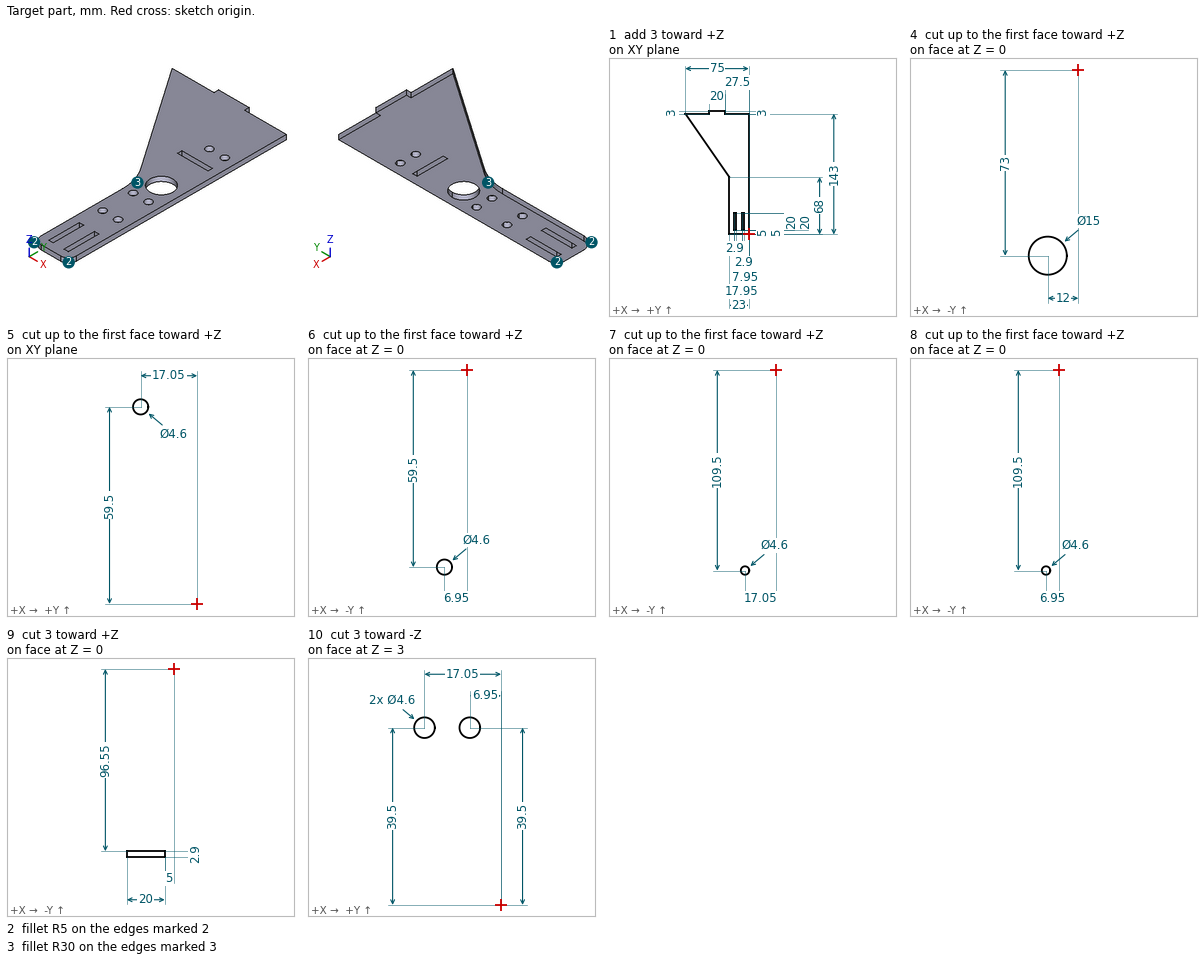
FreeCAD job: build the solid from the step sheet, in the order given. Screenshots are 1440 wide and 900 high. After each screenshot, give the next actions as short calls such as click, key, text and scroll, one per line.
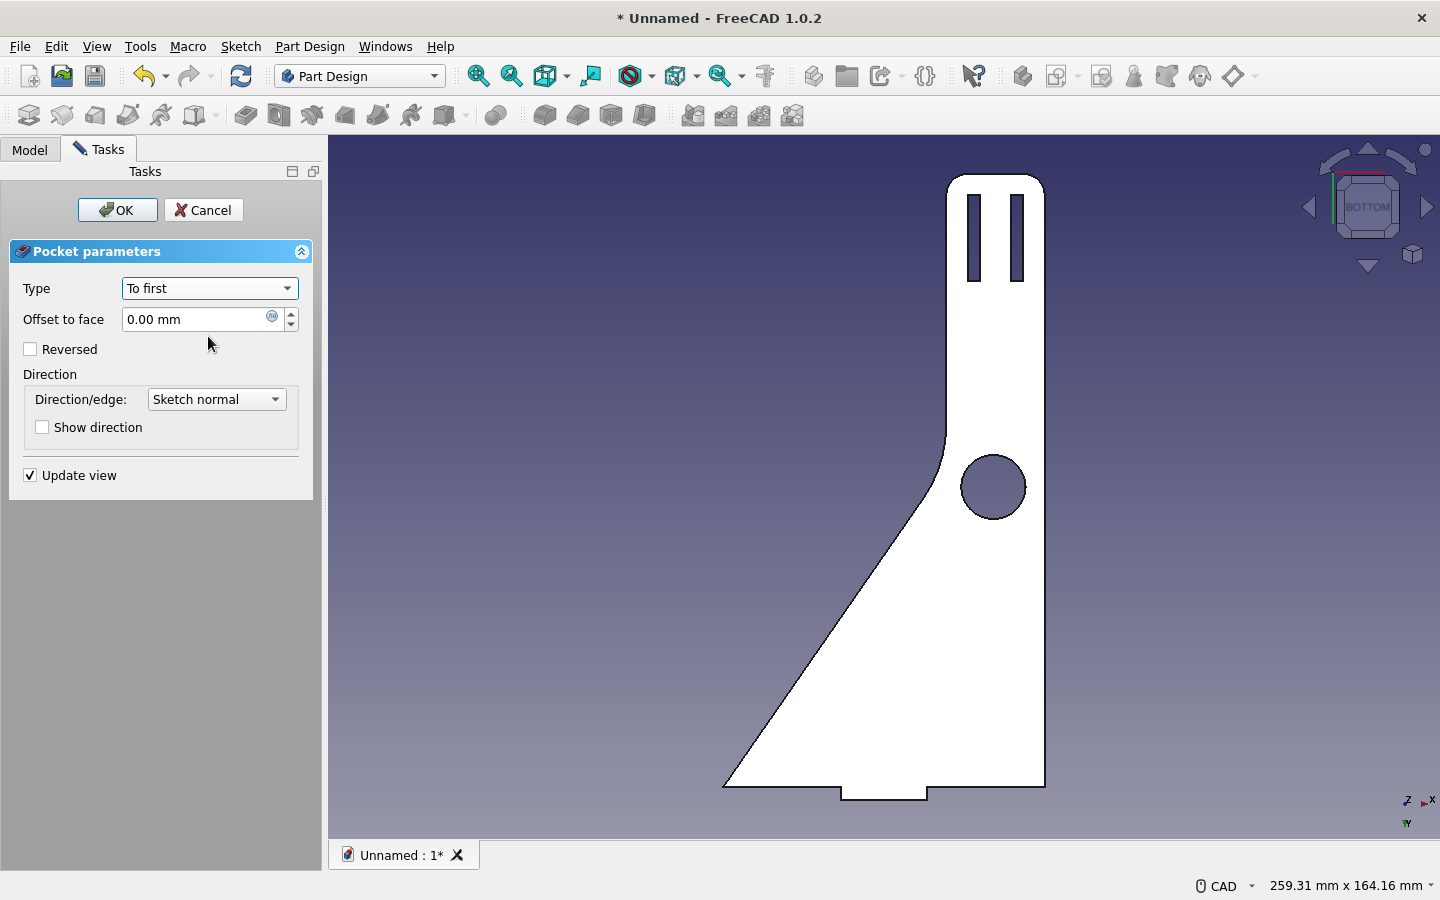
click(118, 210)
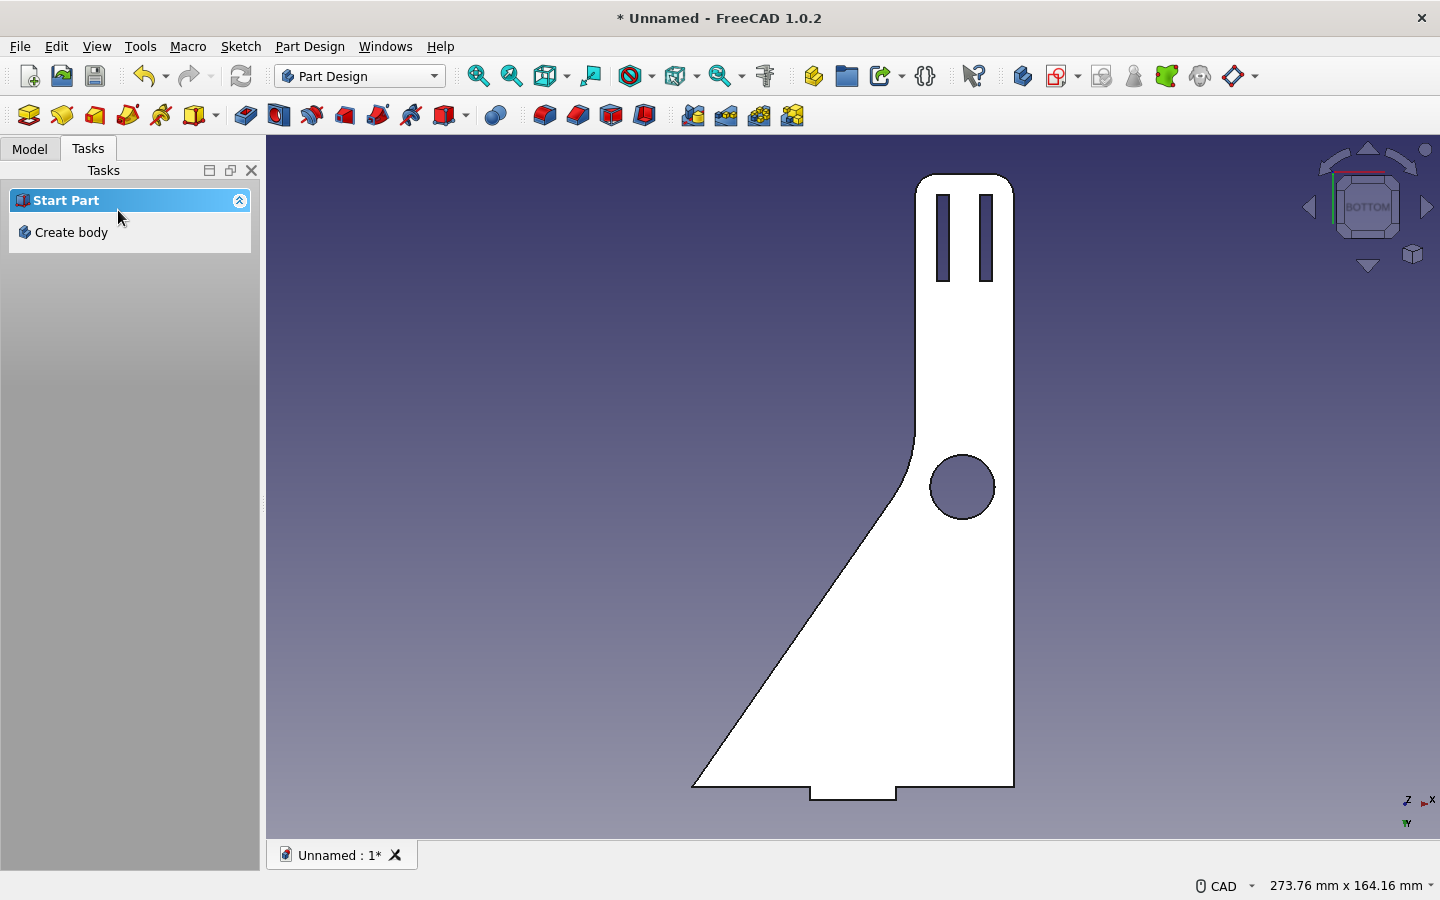
click(1056, 76)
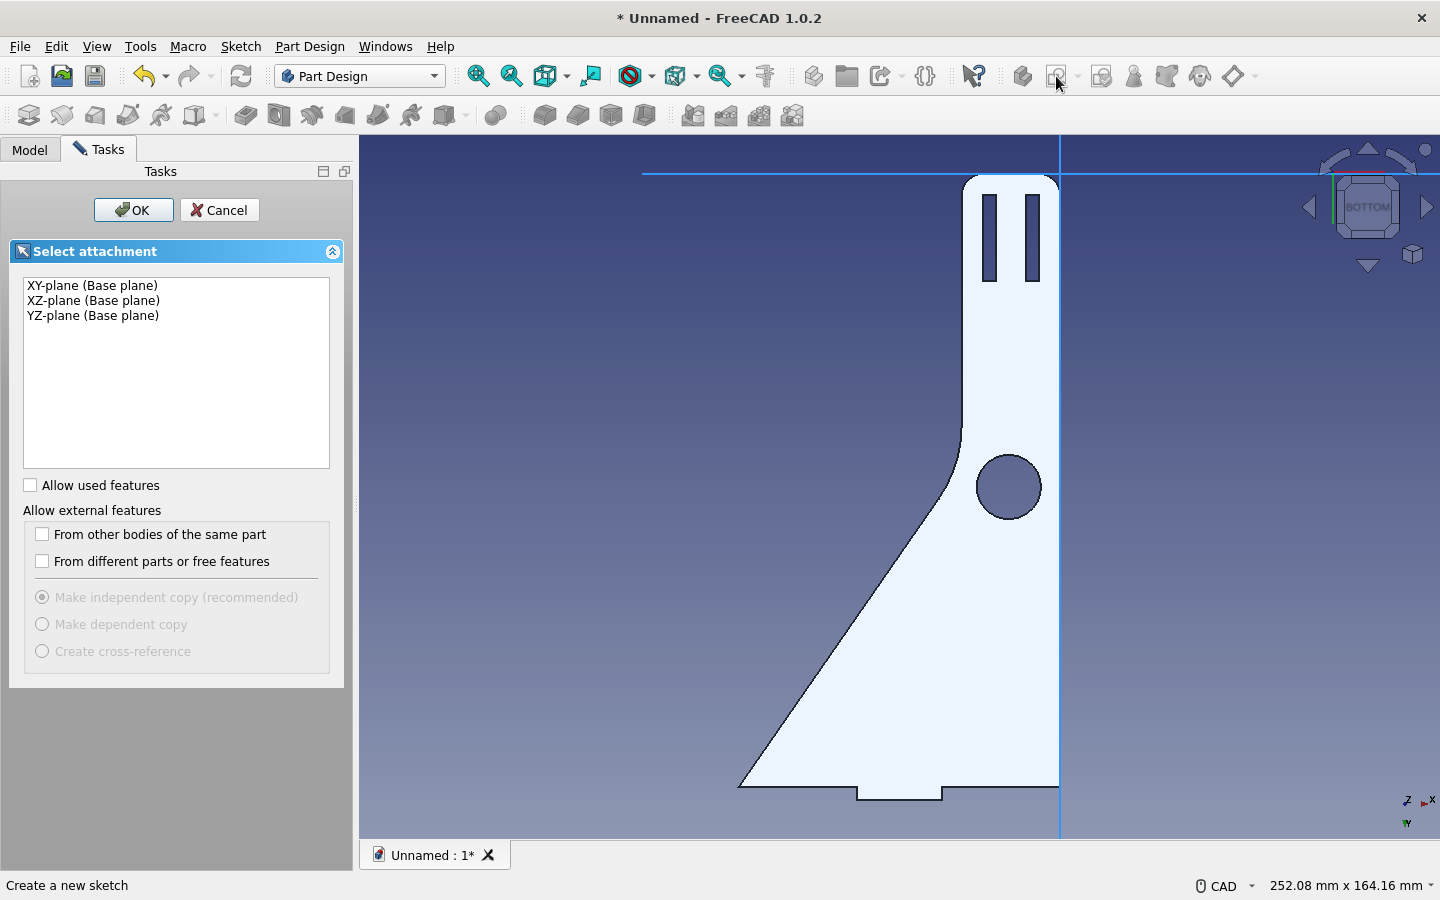
click(84, 286)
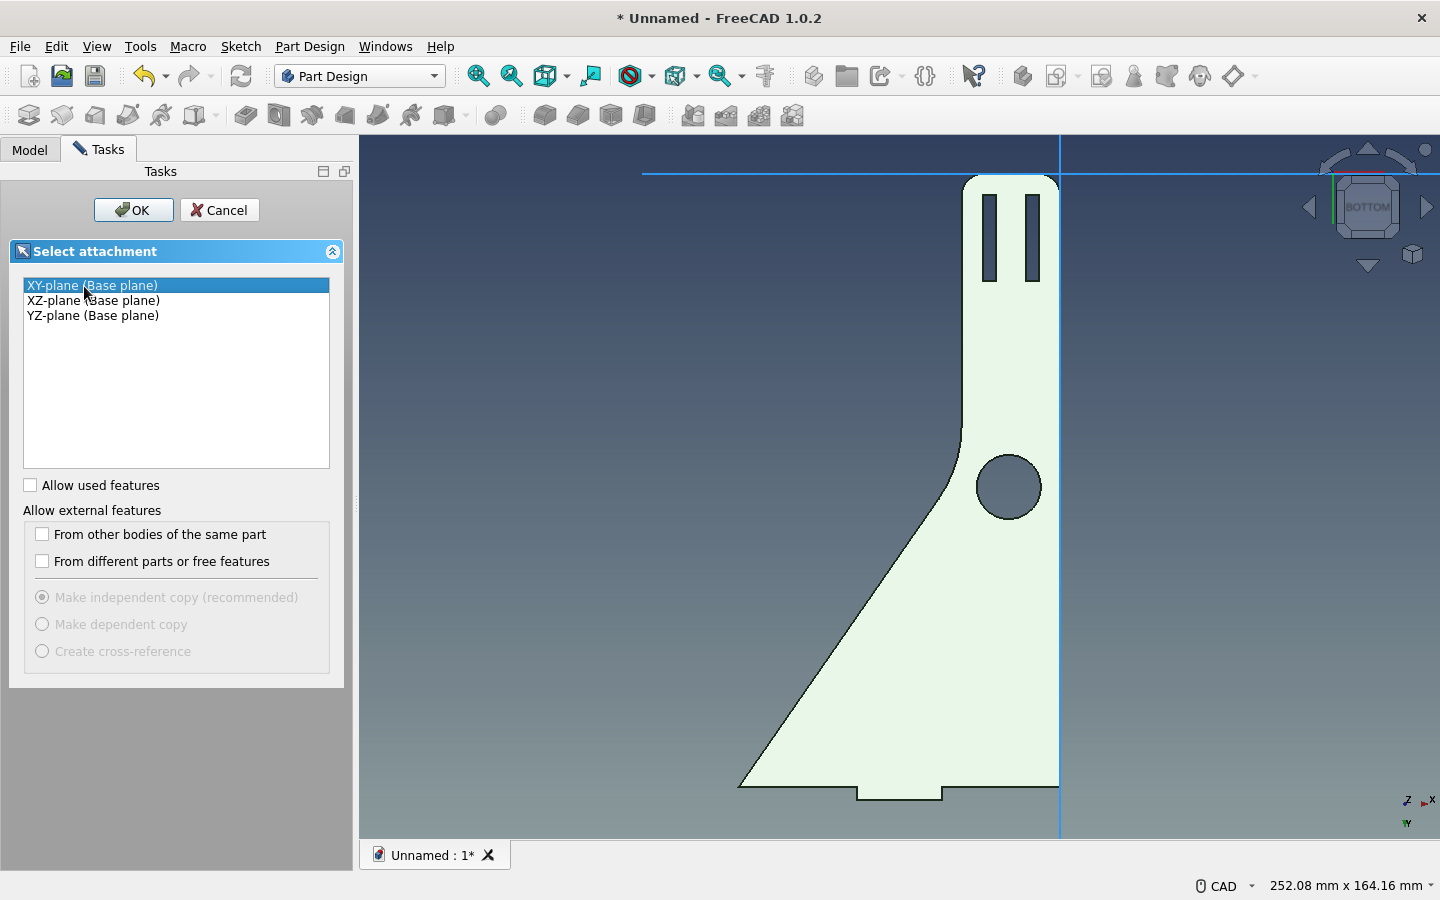
click(134, 210)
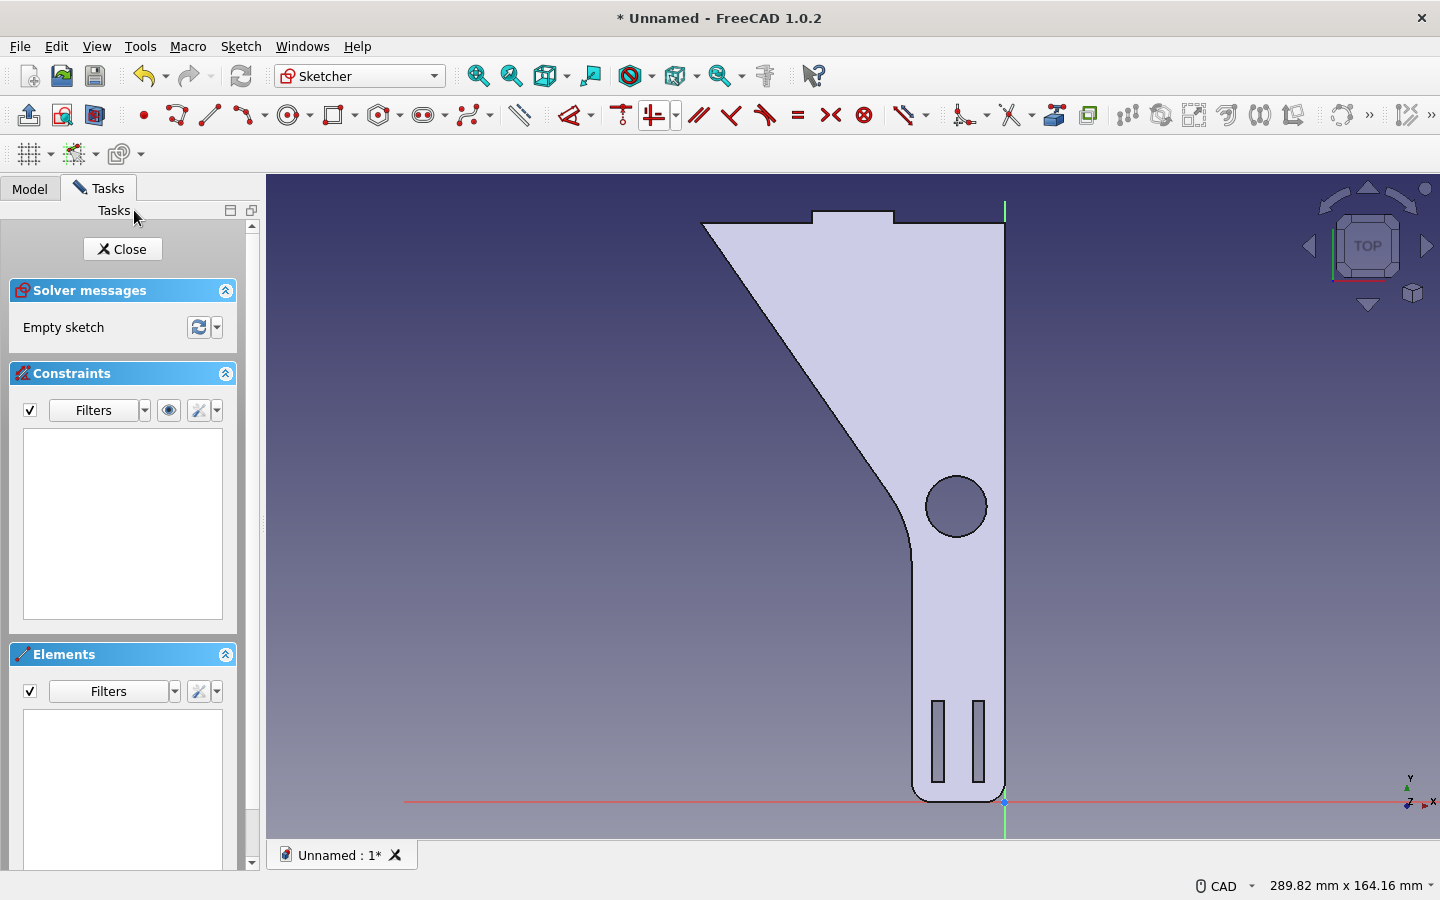
key(q)
key(s)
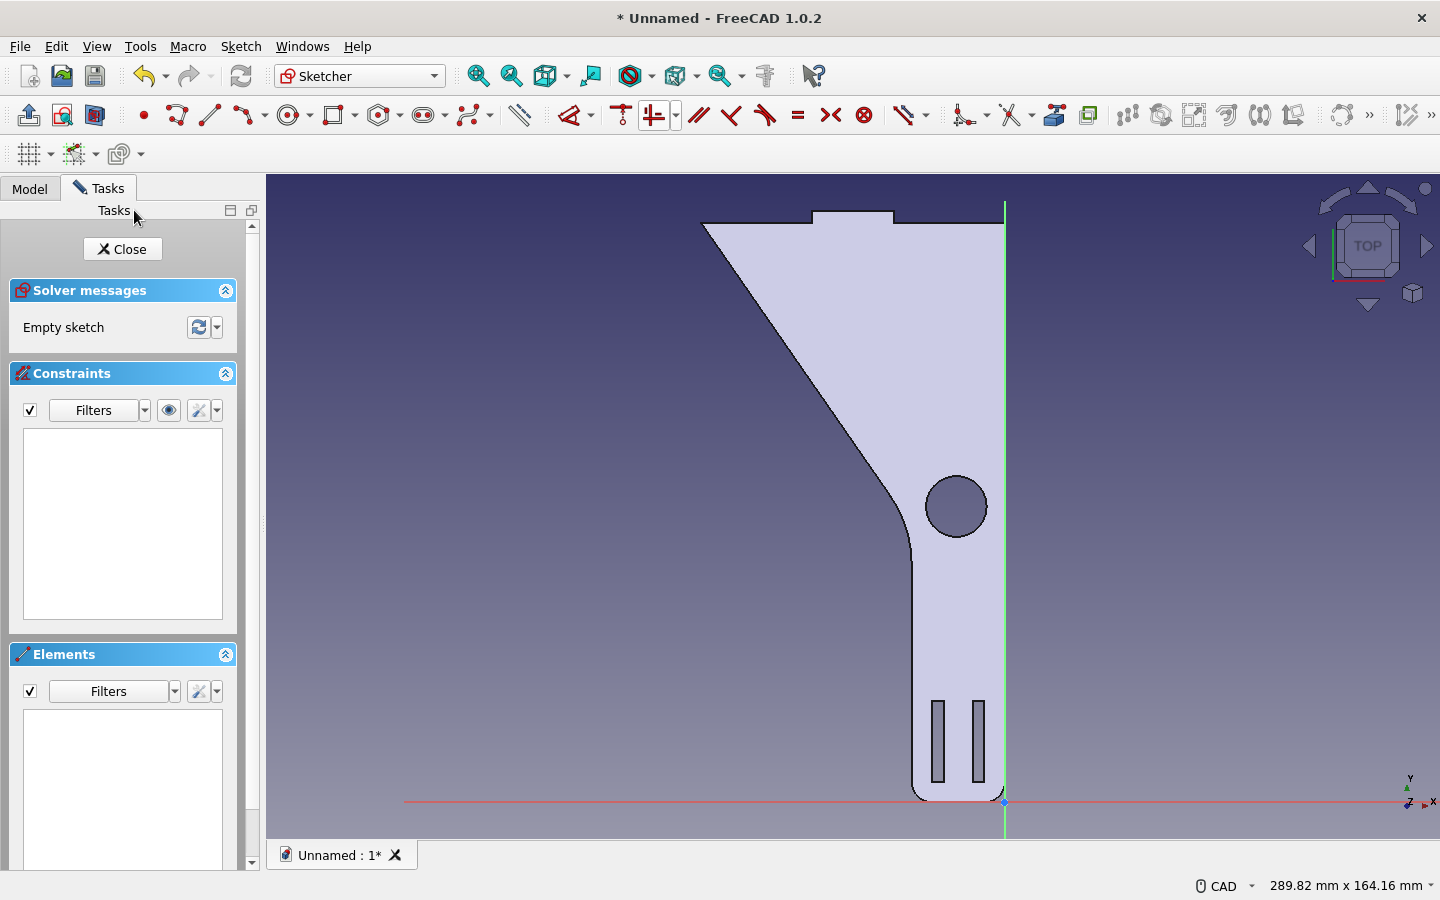
scroll(944, 564, up, 15)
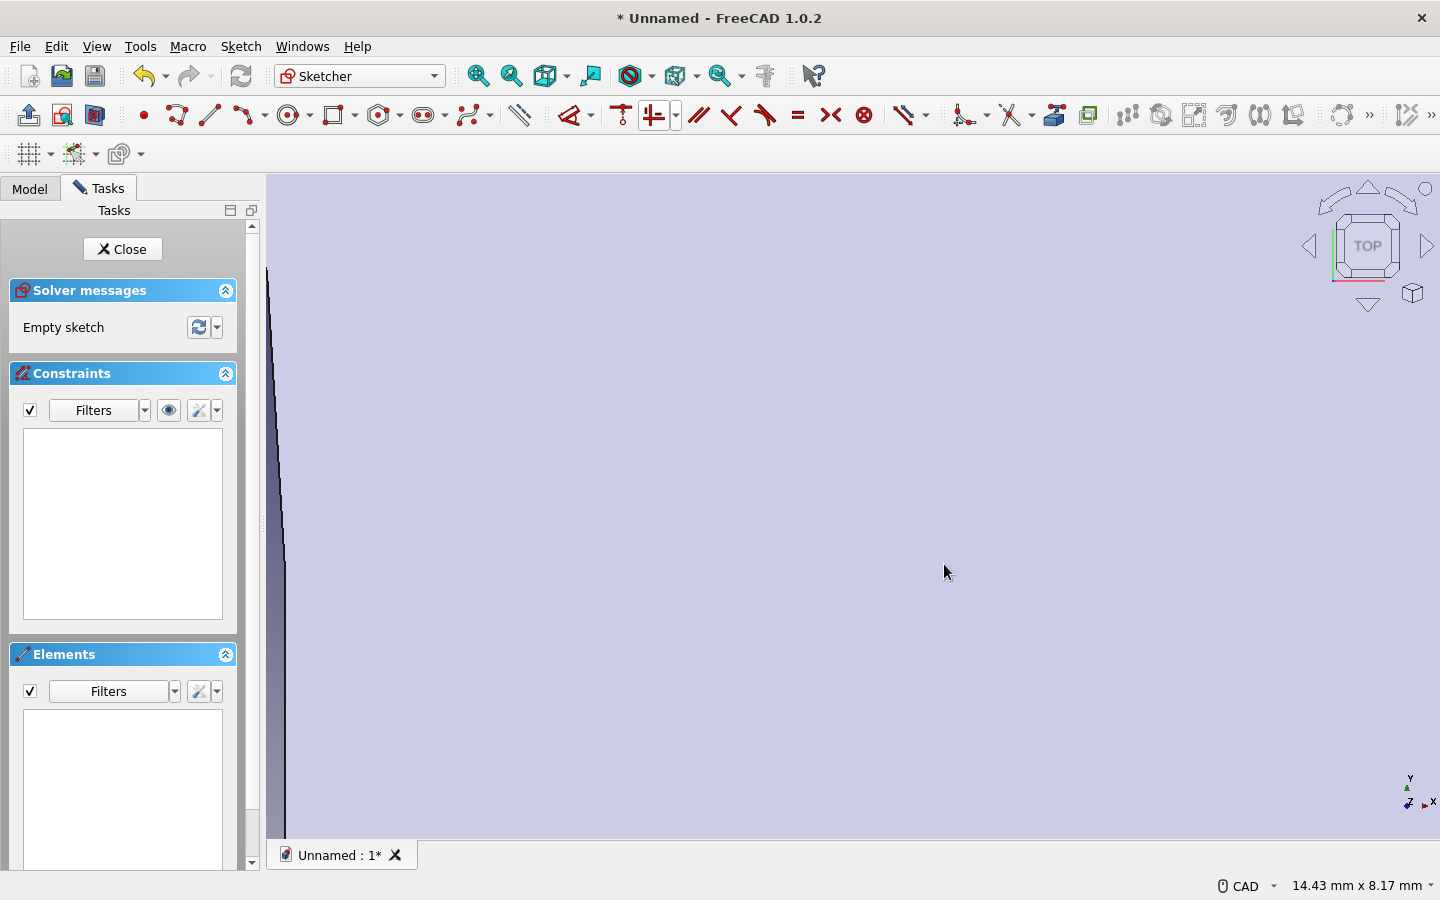
click(288, 116)